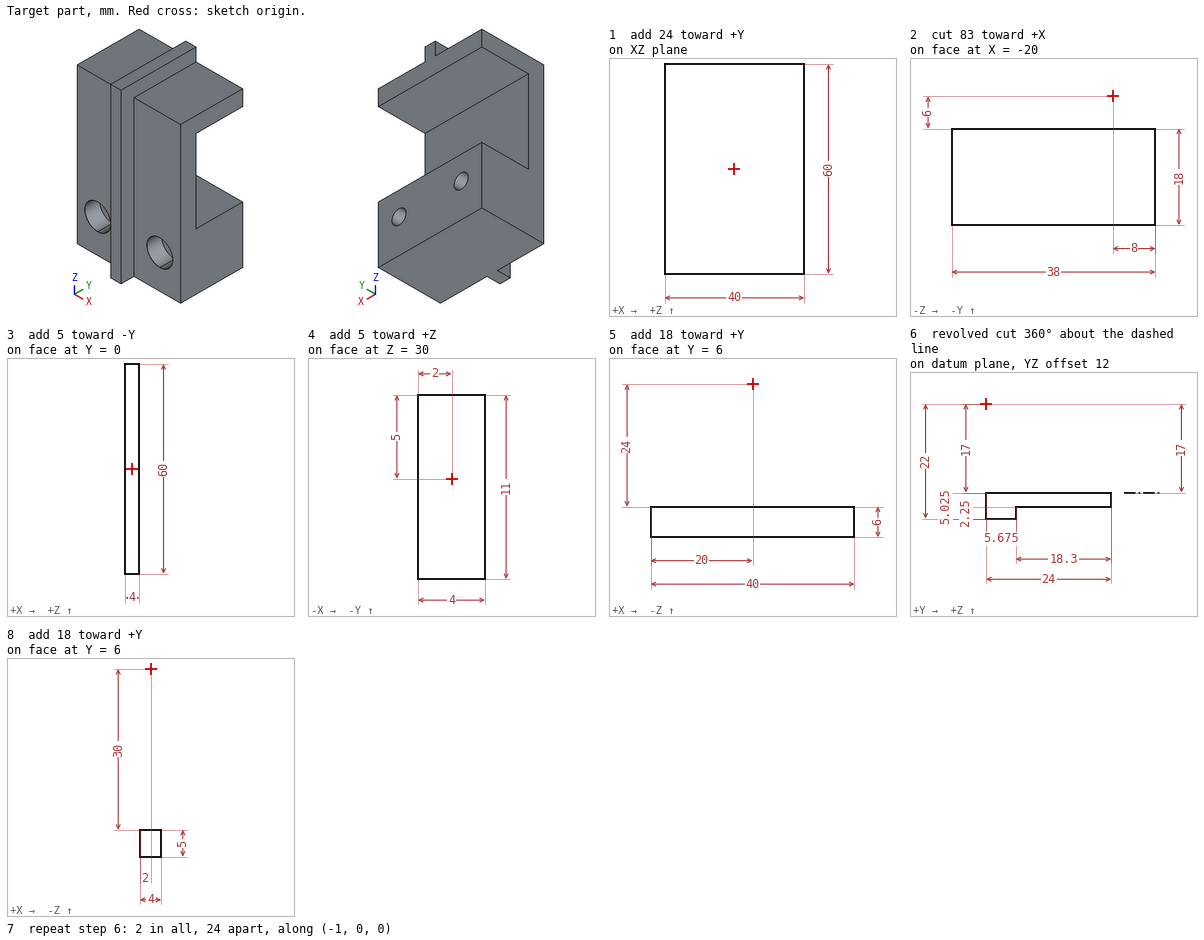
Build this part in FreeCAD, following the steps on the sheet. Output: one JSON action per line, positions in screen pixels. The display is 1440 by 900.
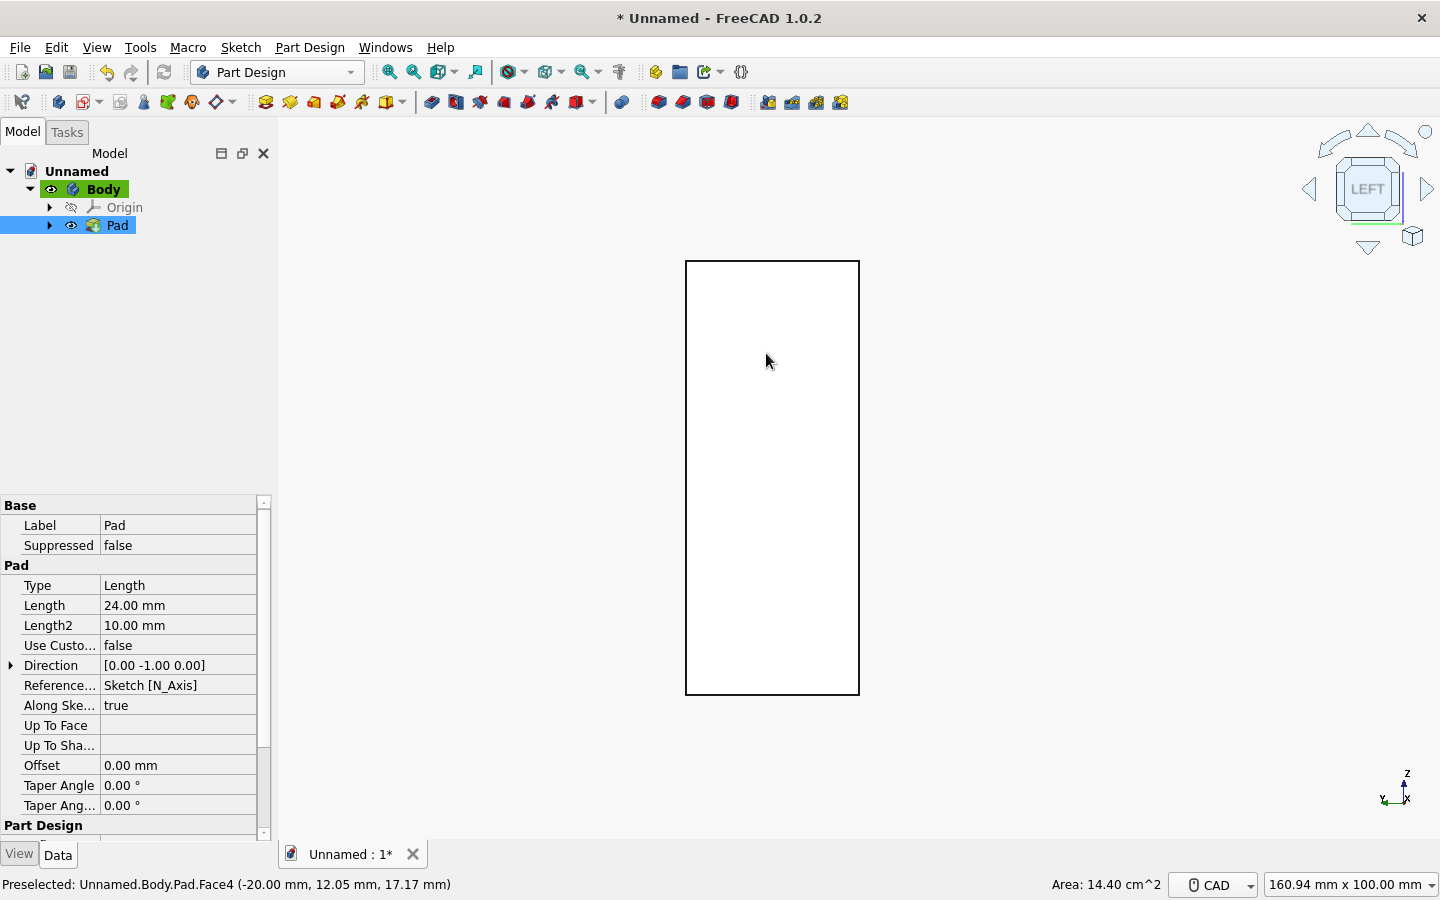
{"action": "left_click", "coordinate": [84, 102]}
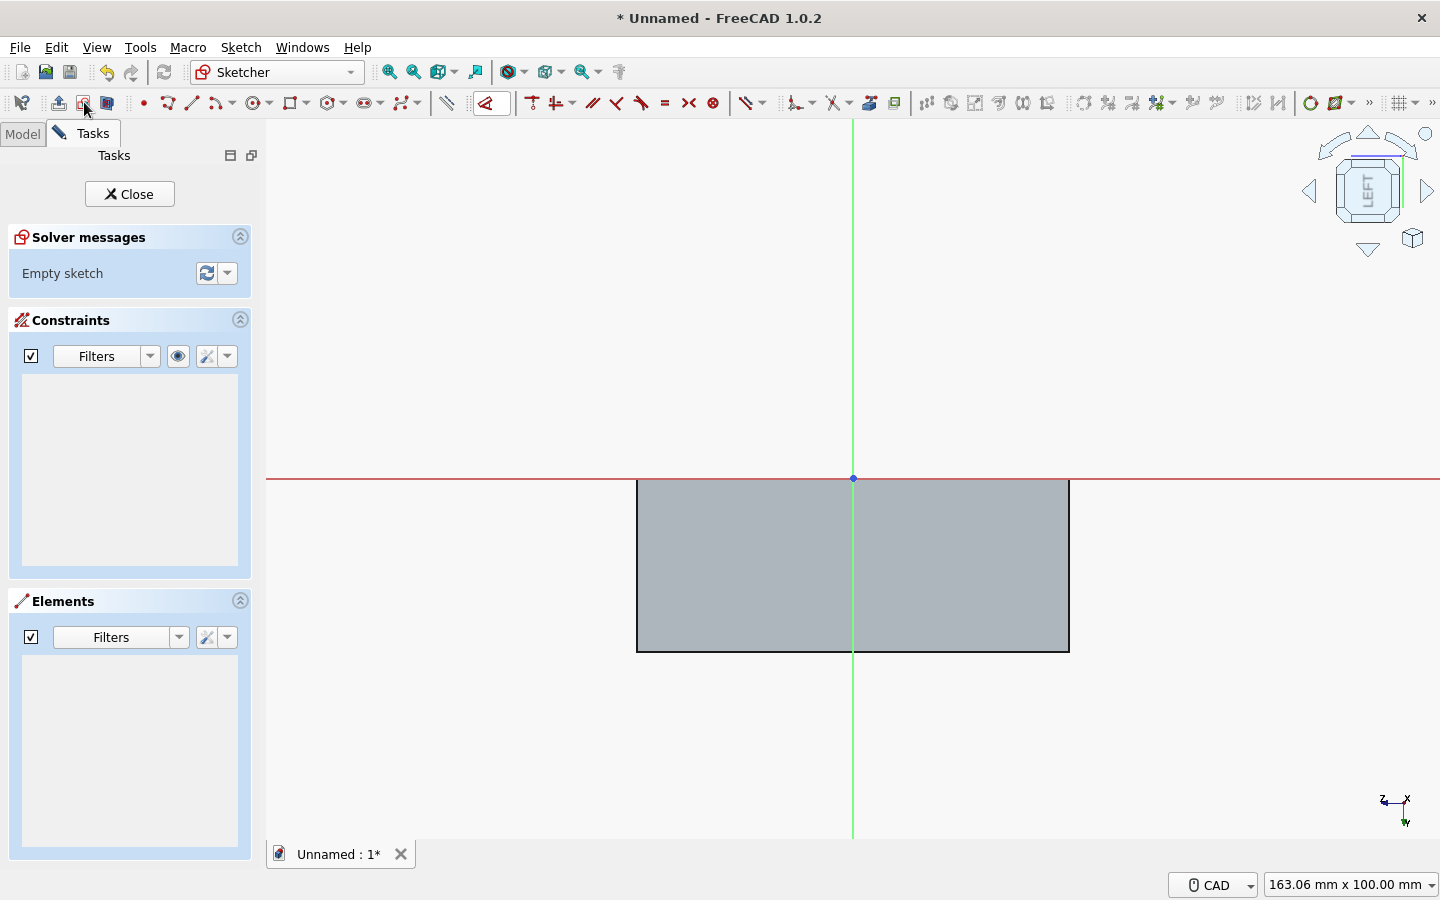
{"action": "scroll", "coordinate": [768, 616], "scroll_direction": "up", "scroll_amount": 5}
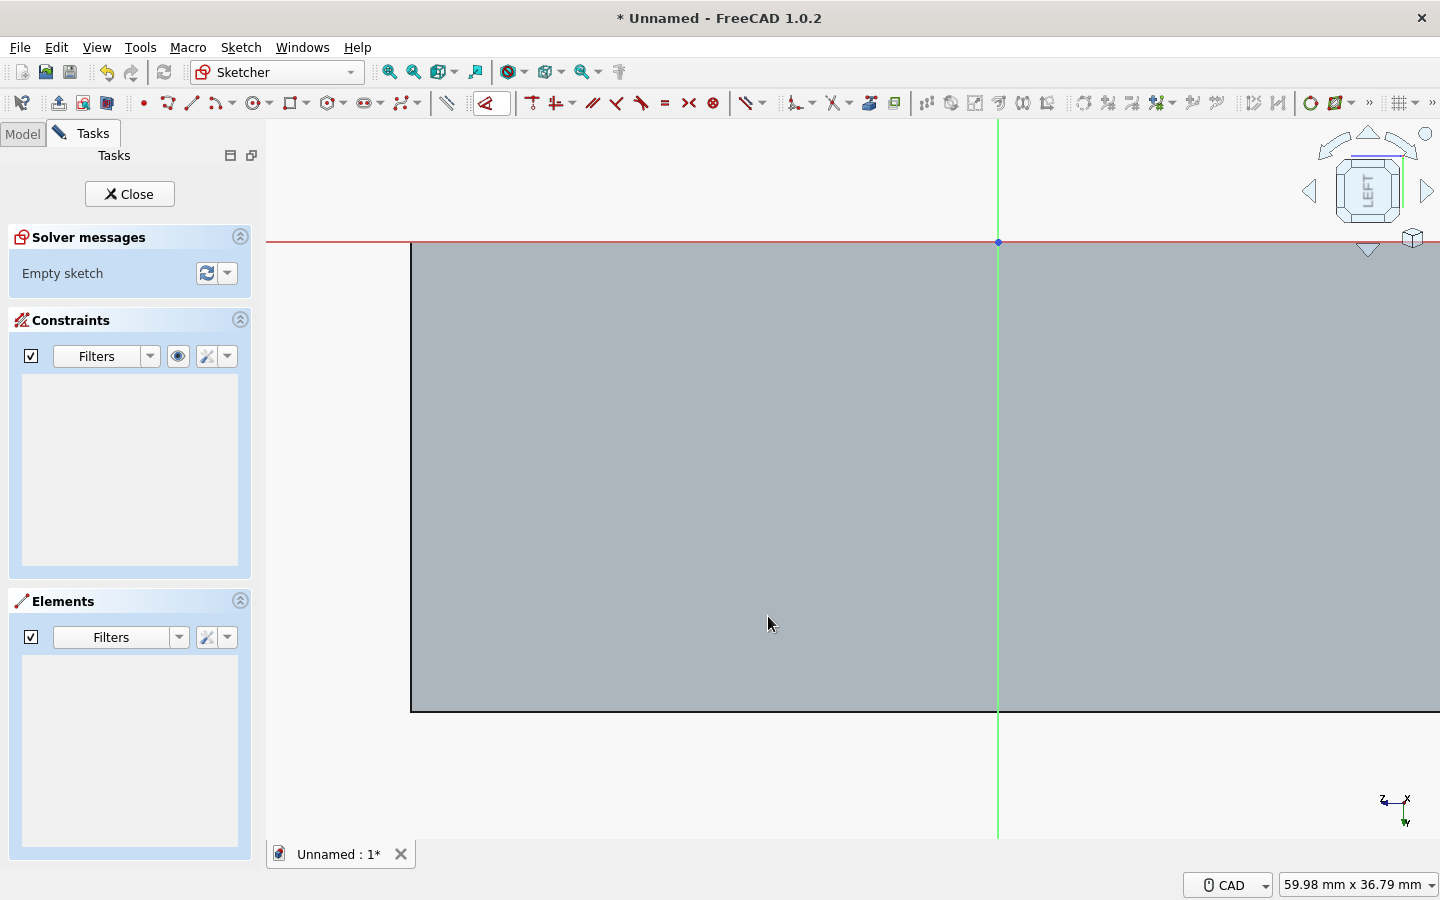
{"action": "key", "text": "g r"}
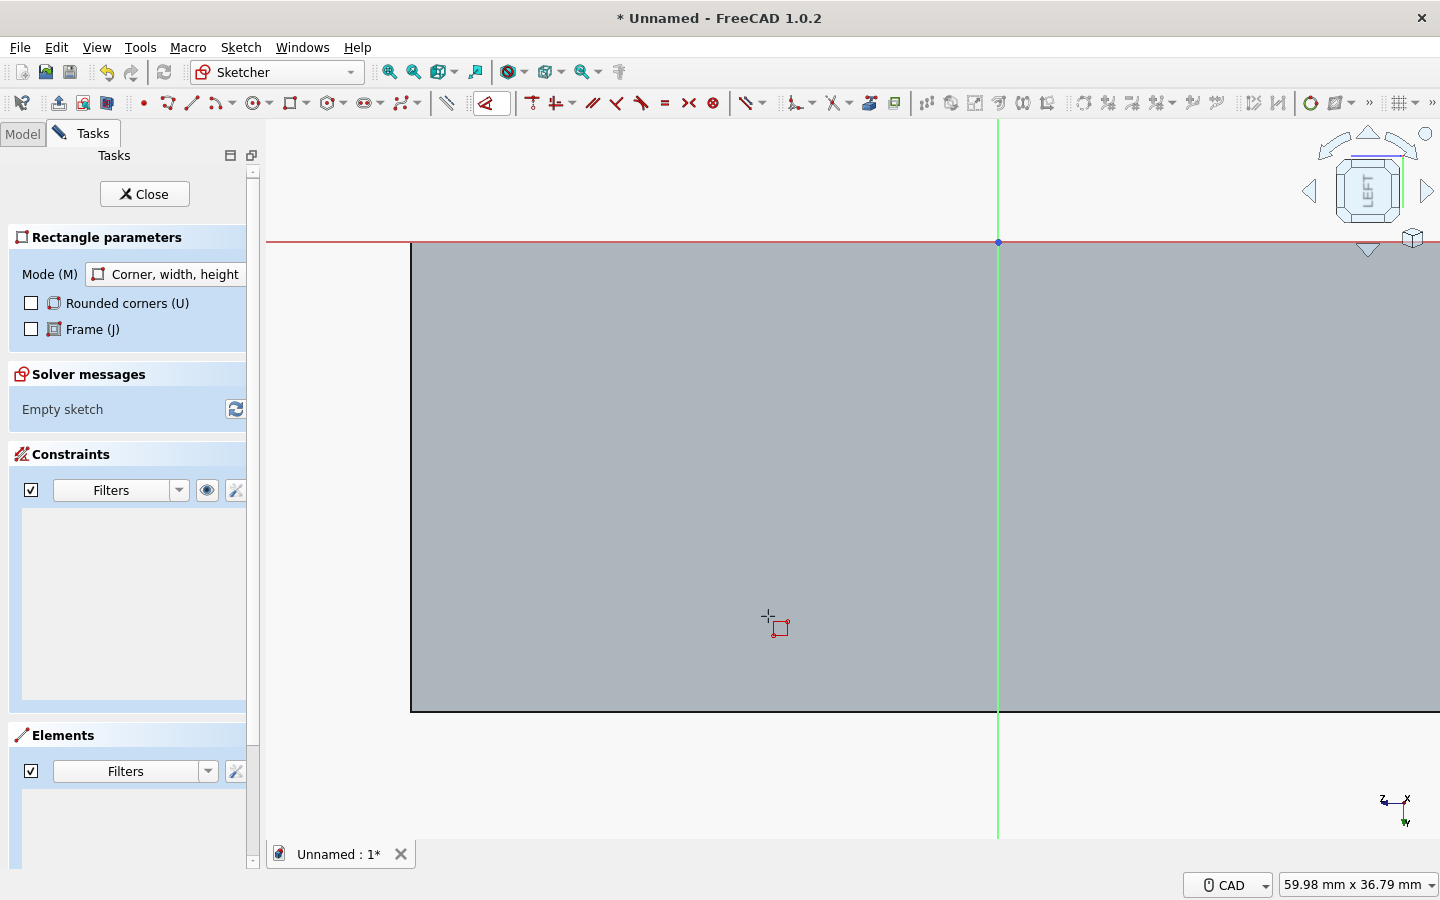
{"action": "left_click", "coordinate": [411, 360]}
{"action": "mouse_move", "coordinate": [1155, 712]}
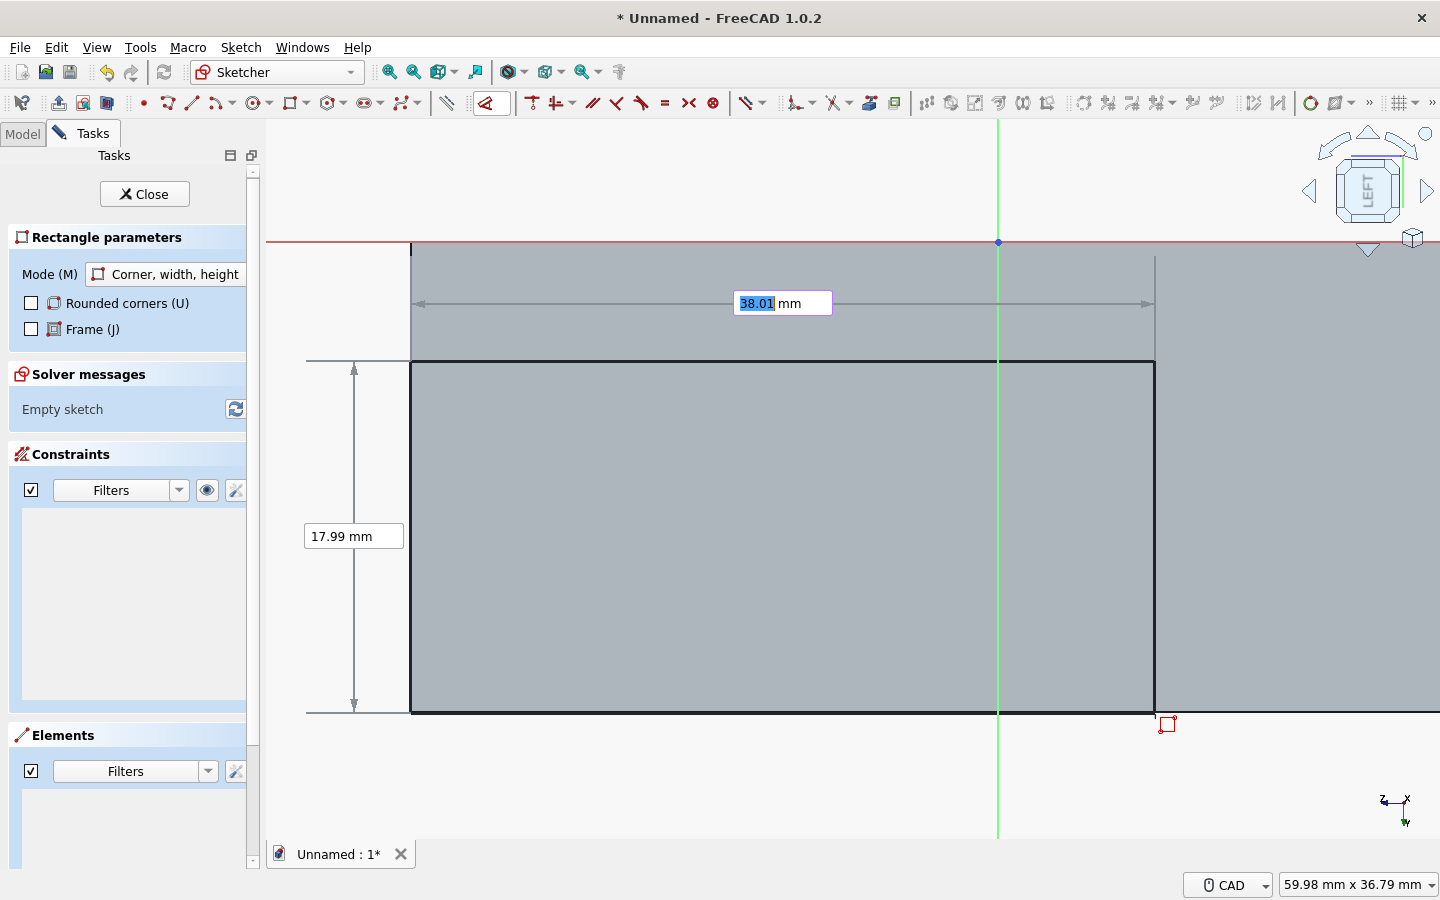
{"action": "type", "text": "38"}
{"action": "key", "text": "Tab"}
{"action": "type", "text": "18"}
{"action": "key", "text": "Return"}
{"action": "key", "text": "Escape"}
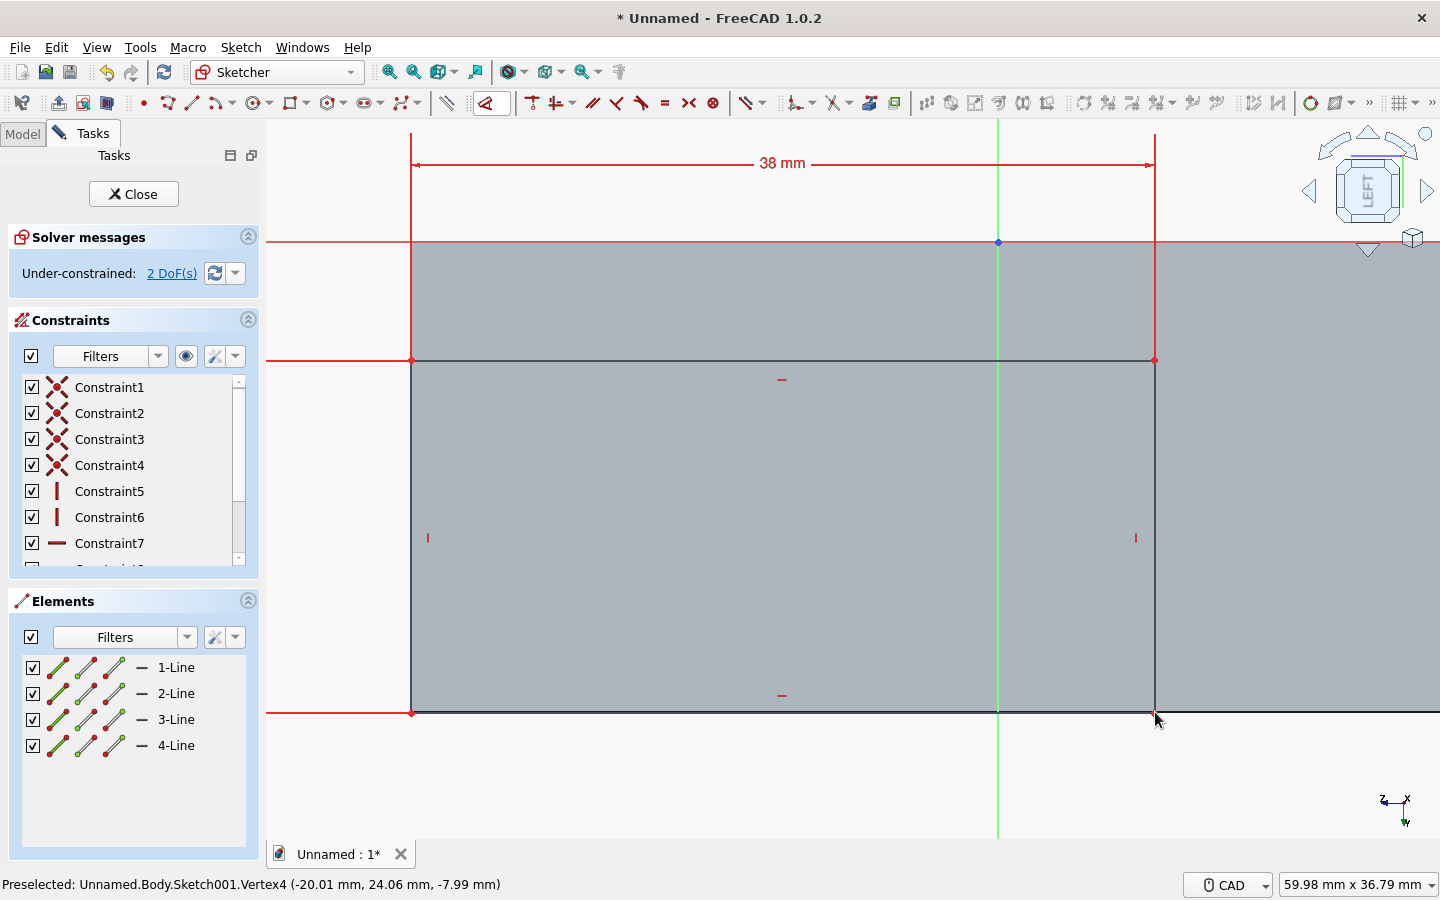
{"action": "key", "text": "d"}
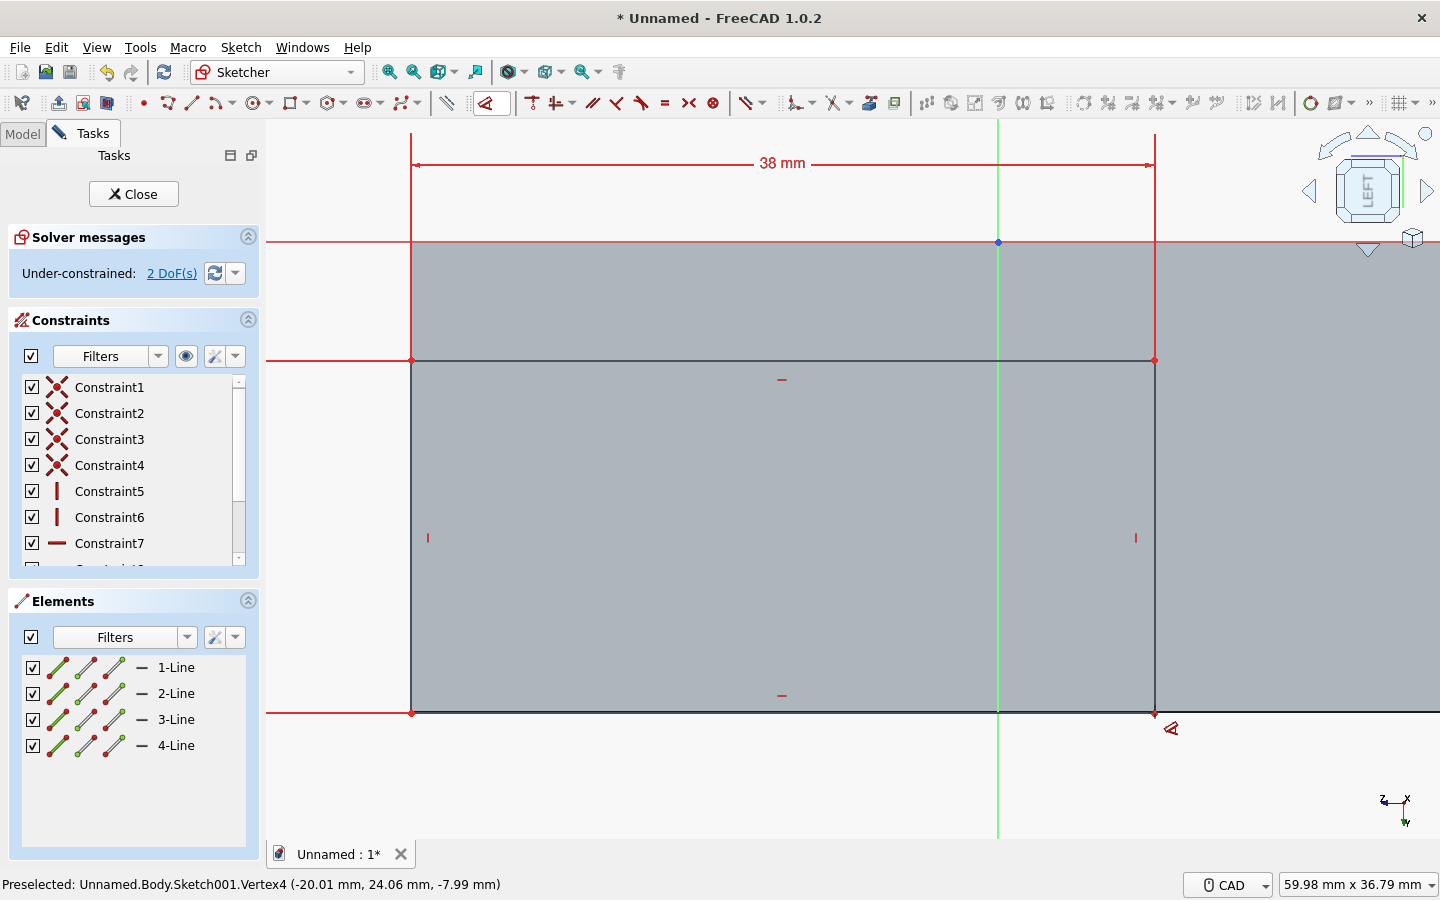
{"action": "left_click", "coordinate": [411, 361]}
{"action": "left_click", "coordinate": [377, 302]}